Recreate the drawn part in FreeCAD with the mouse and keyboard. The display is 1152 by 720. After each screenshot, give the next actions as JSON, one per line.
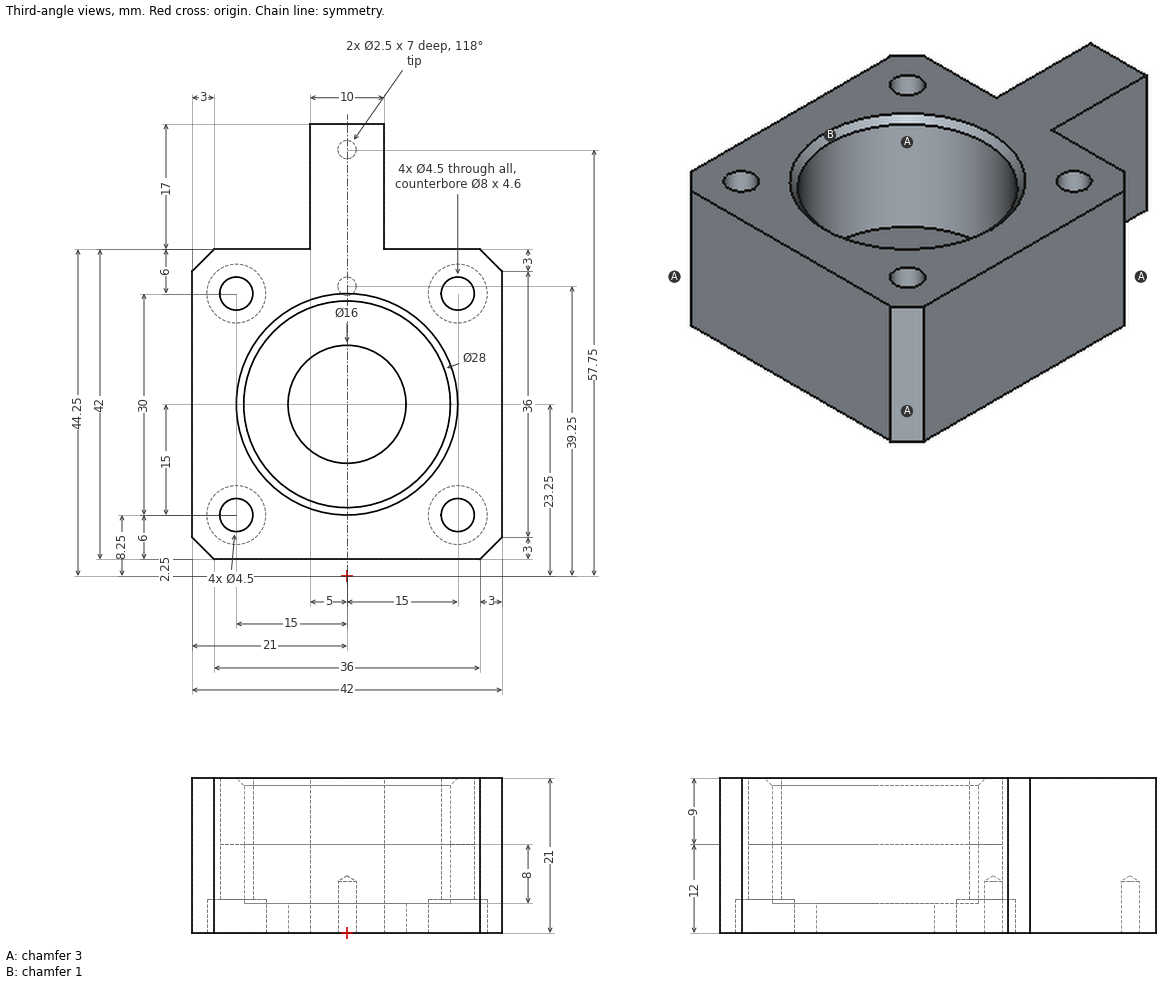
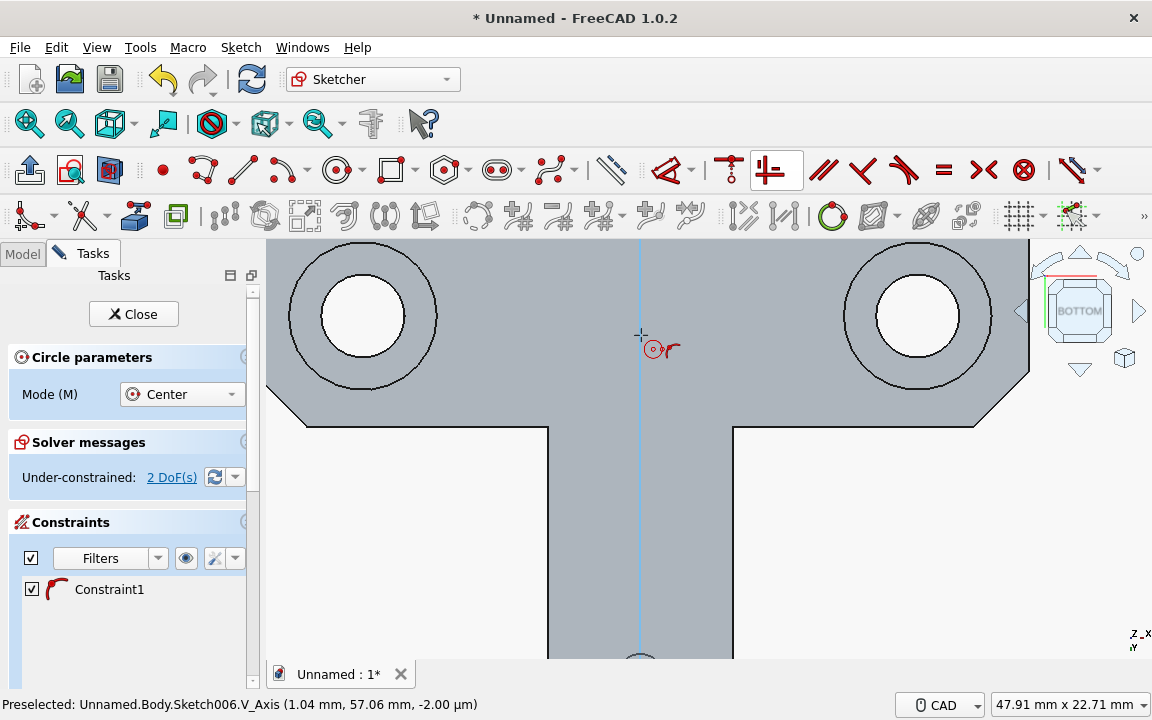
{"action": "left_click", "coordinate": [640, 334]}
{"action": "left_click", "coordinate": [657, 318]}
{"action": "key", "text": "Escape"}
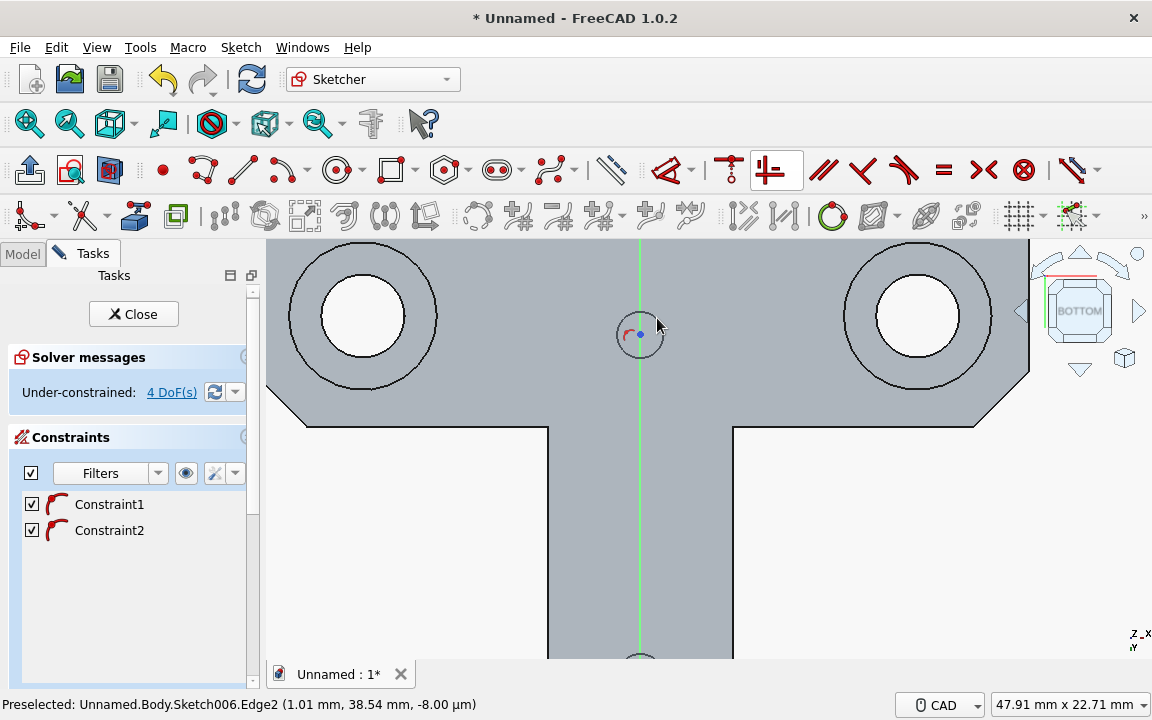
{"action": "scroll", "coordinate": [641, 334], "scroll_direction": "down", "scroll_amount": 2}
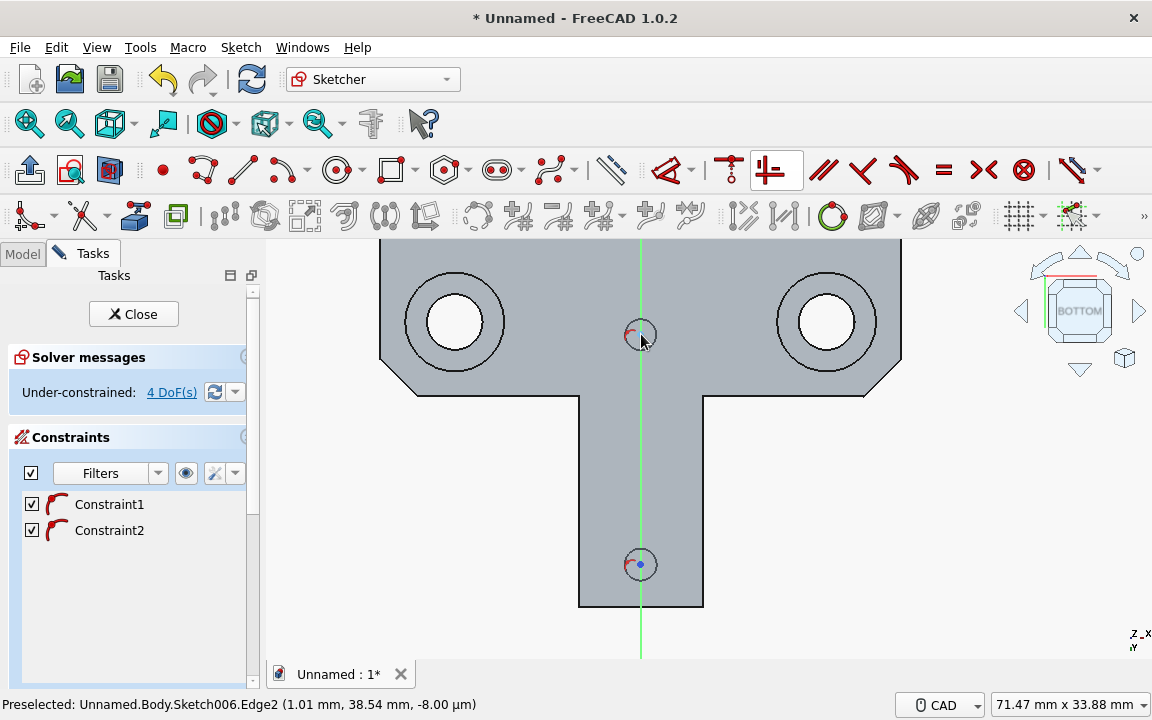
{"action": "scroll", "coordinate": [652, 553], "scroll_direction": "up", "scroll_amount": 2}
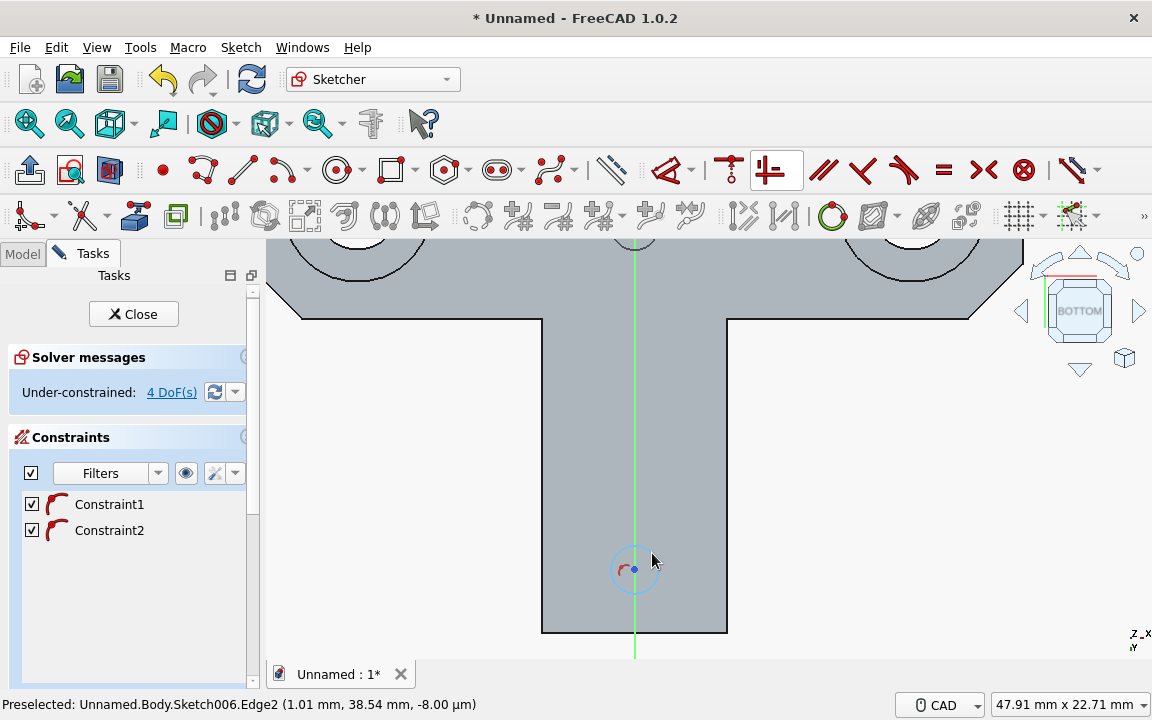
{"action": "left_click", "coordinate": [652, 553]}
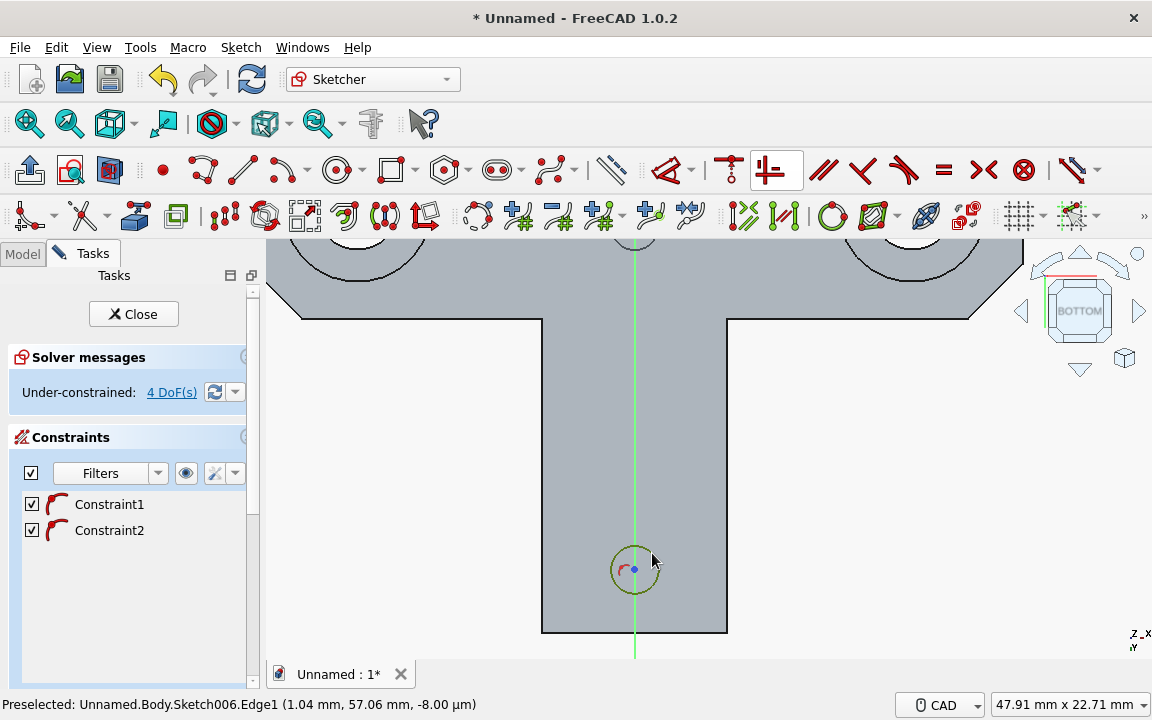
{"action": "scroll", "coordinate": [652, 554], "scroll_direction": "down", "scroll_amount": 2}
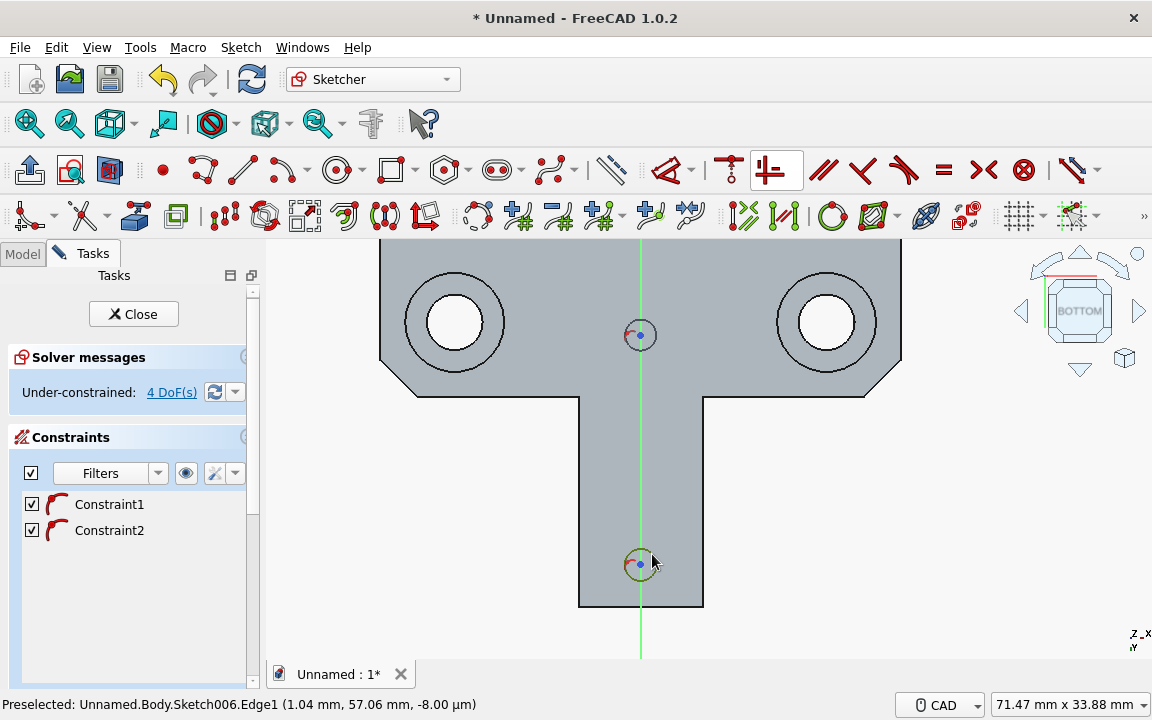
{"action": "scroll", "coordinate": [652, 324], "scroll_direction": "up", "scroll_amount": 2}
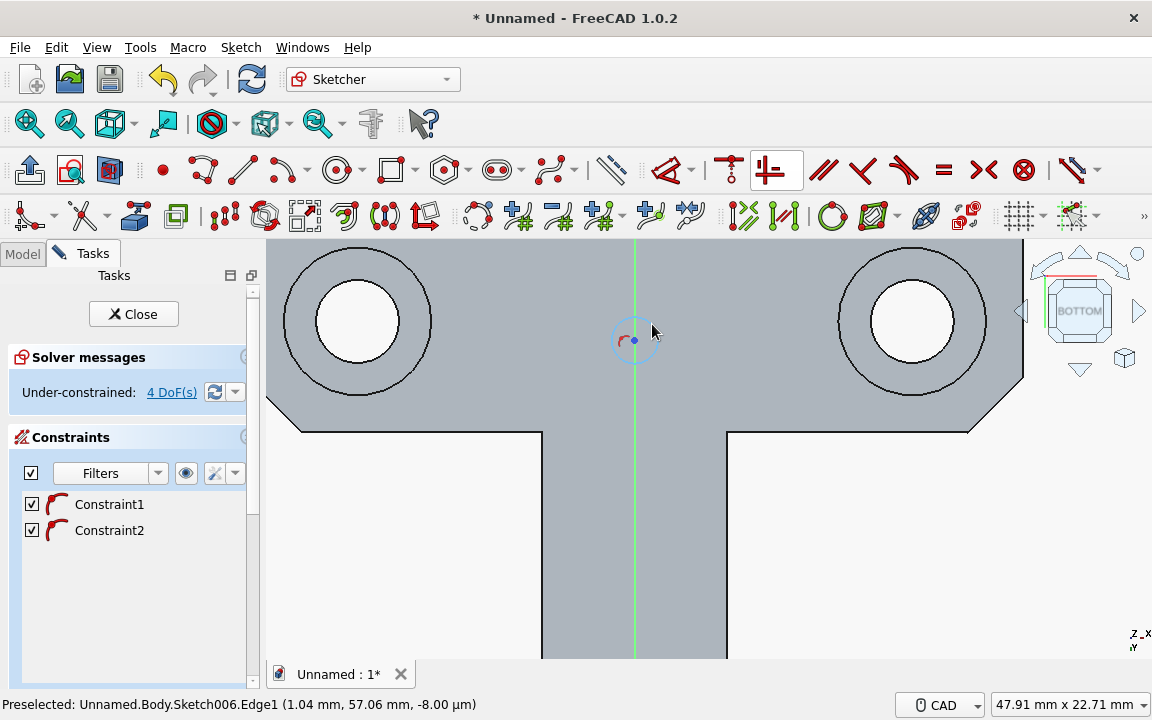
{"action": "left_click", "coordinate": [651, 324]}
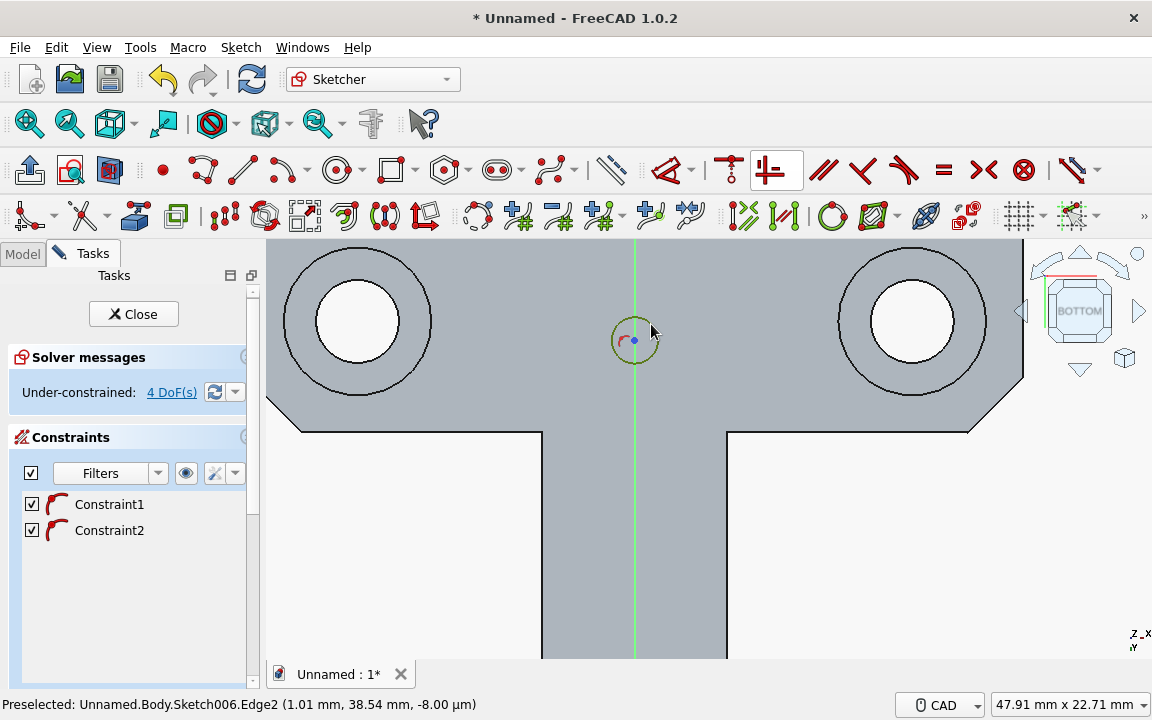
{"action": "left_click", "coordinate": [944, 170]}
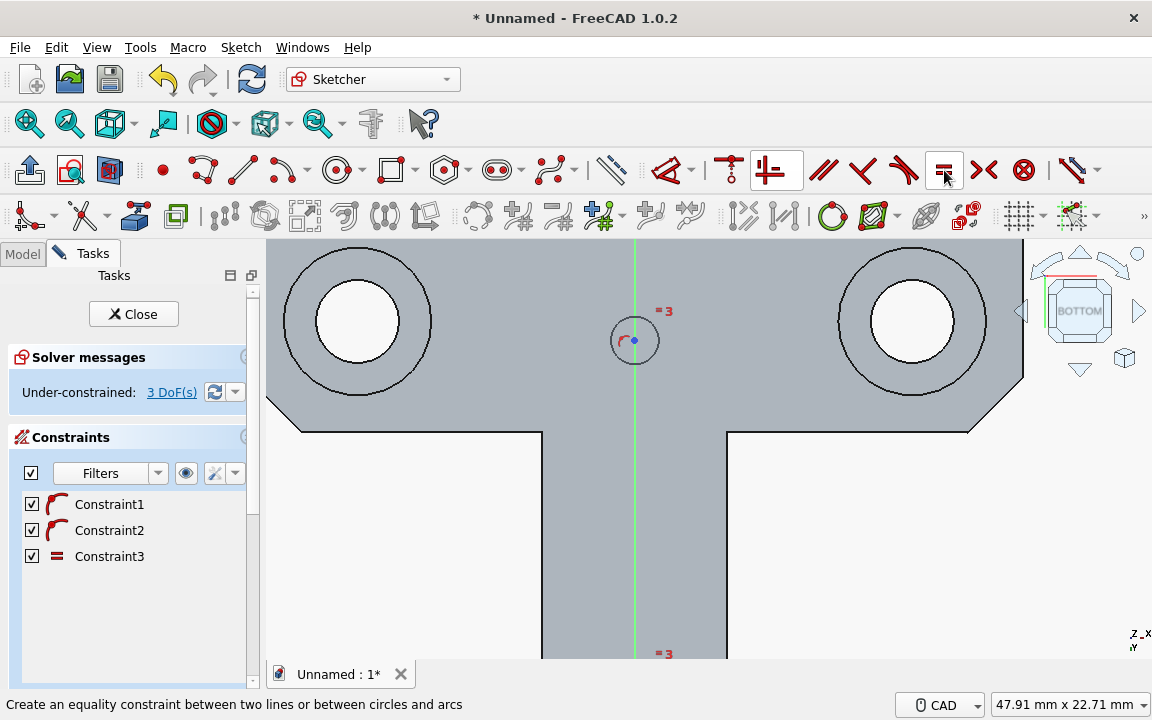
{"action": "left_click", "coordinate": [666, 170]}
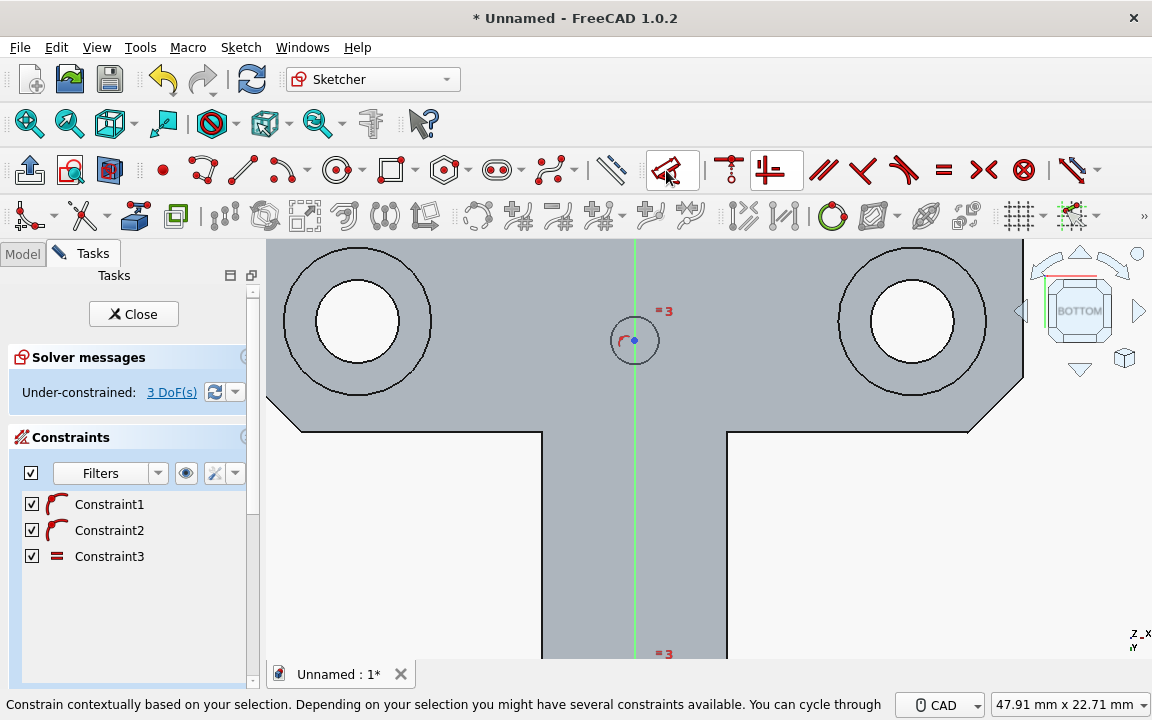
{"action": "scroll", "coordinate": [652, 323], "scroll_direction": "down", "scroll_amount": 2}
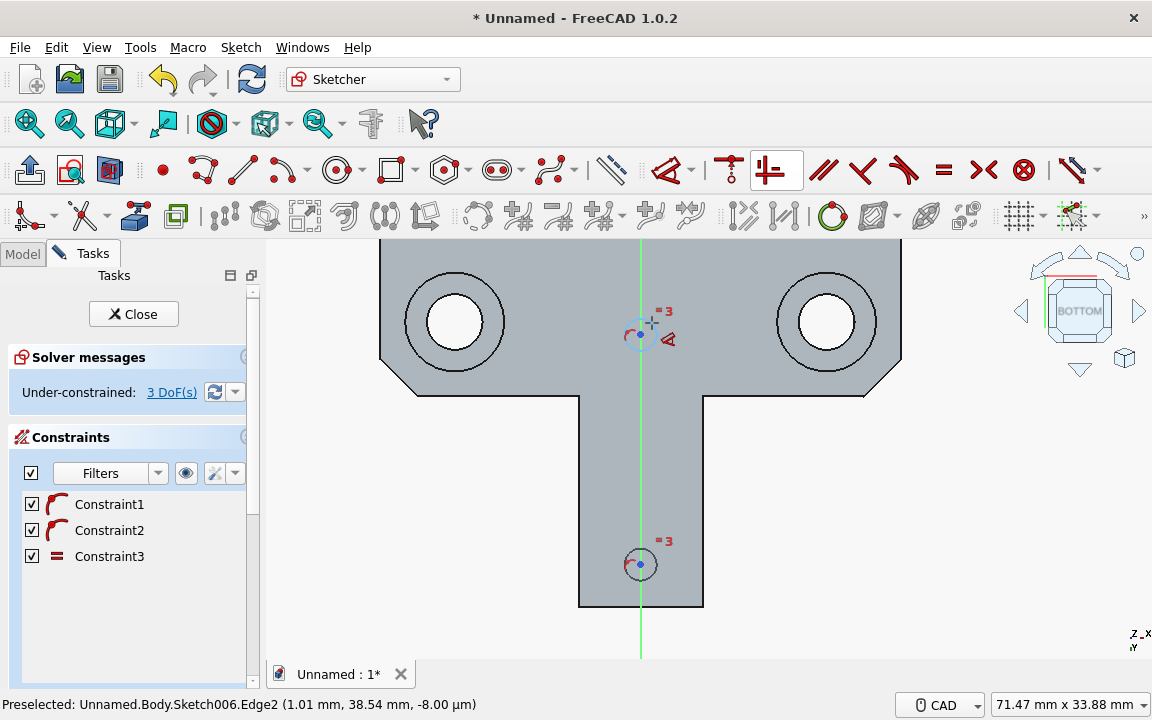
{"action": "scroll", "coordinate": [652, 553], "scroll_direction": "up", "scroll_amount": 2}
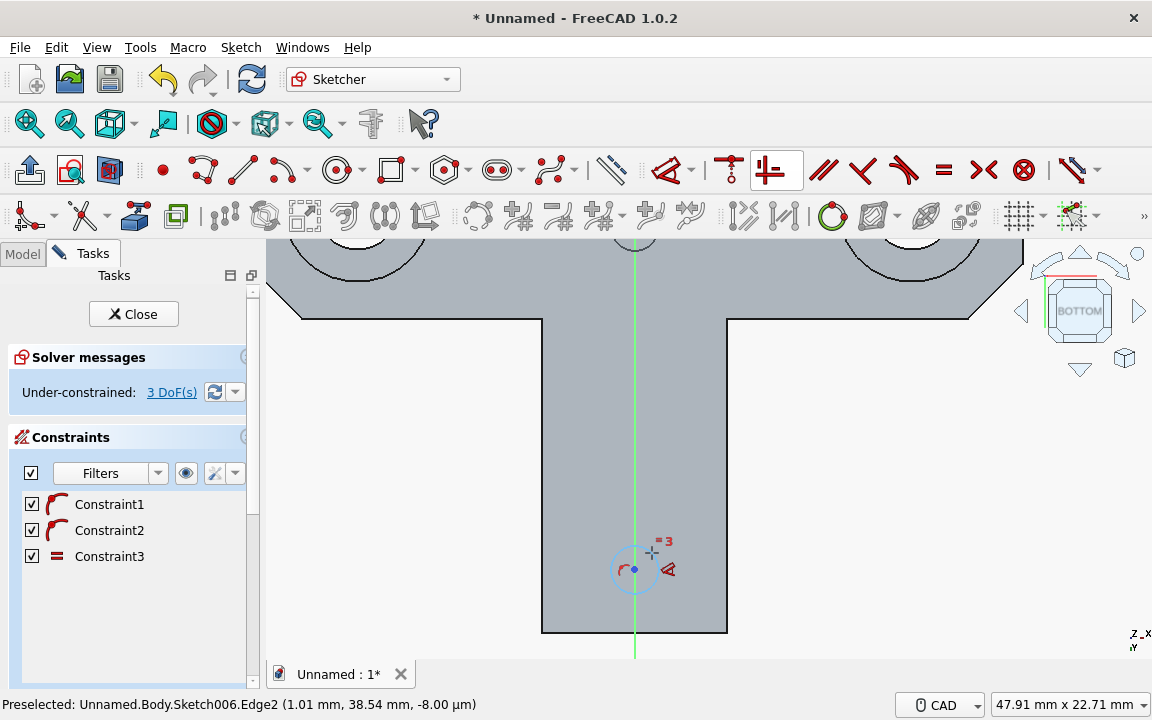
{"action": "left_click", "coordinate": [652, 553]}
{"action": "left_click", "coordinate": [675, 531]}